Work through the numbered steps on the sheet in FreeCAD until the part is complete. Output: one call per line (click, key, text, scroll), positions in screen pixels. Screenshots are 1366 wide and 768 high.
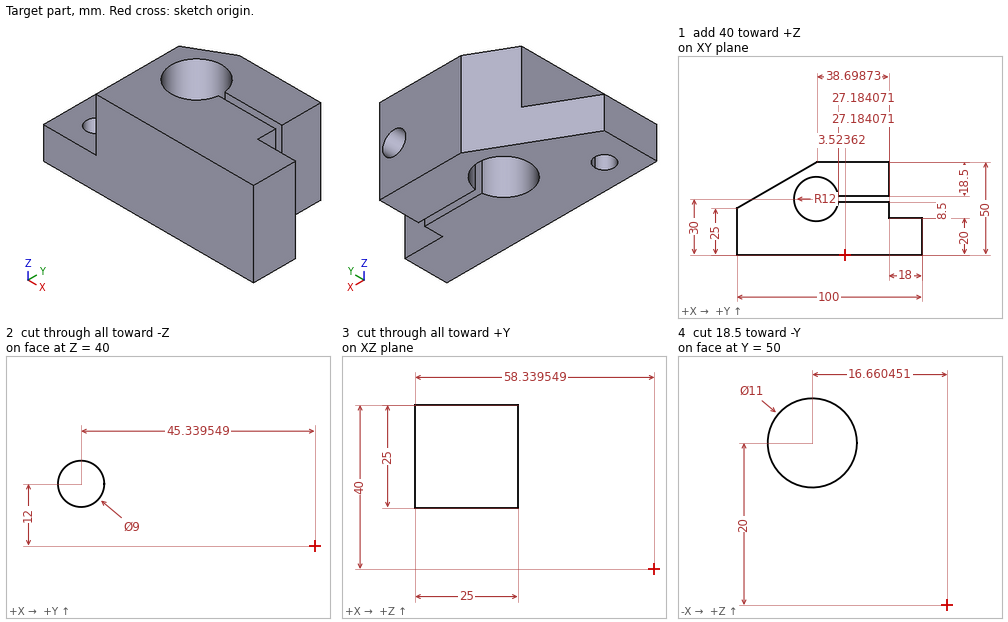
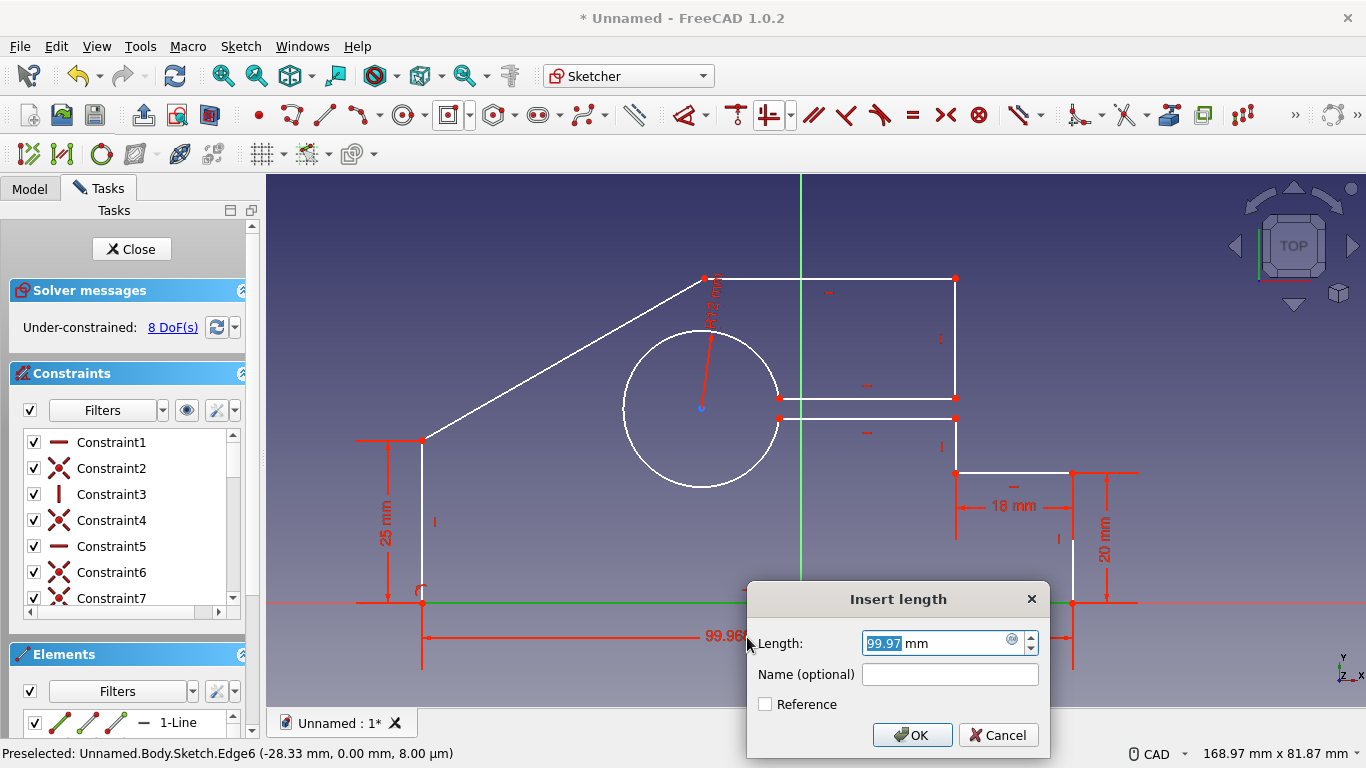
text(100)
key(Return)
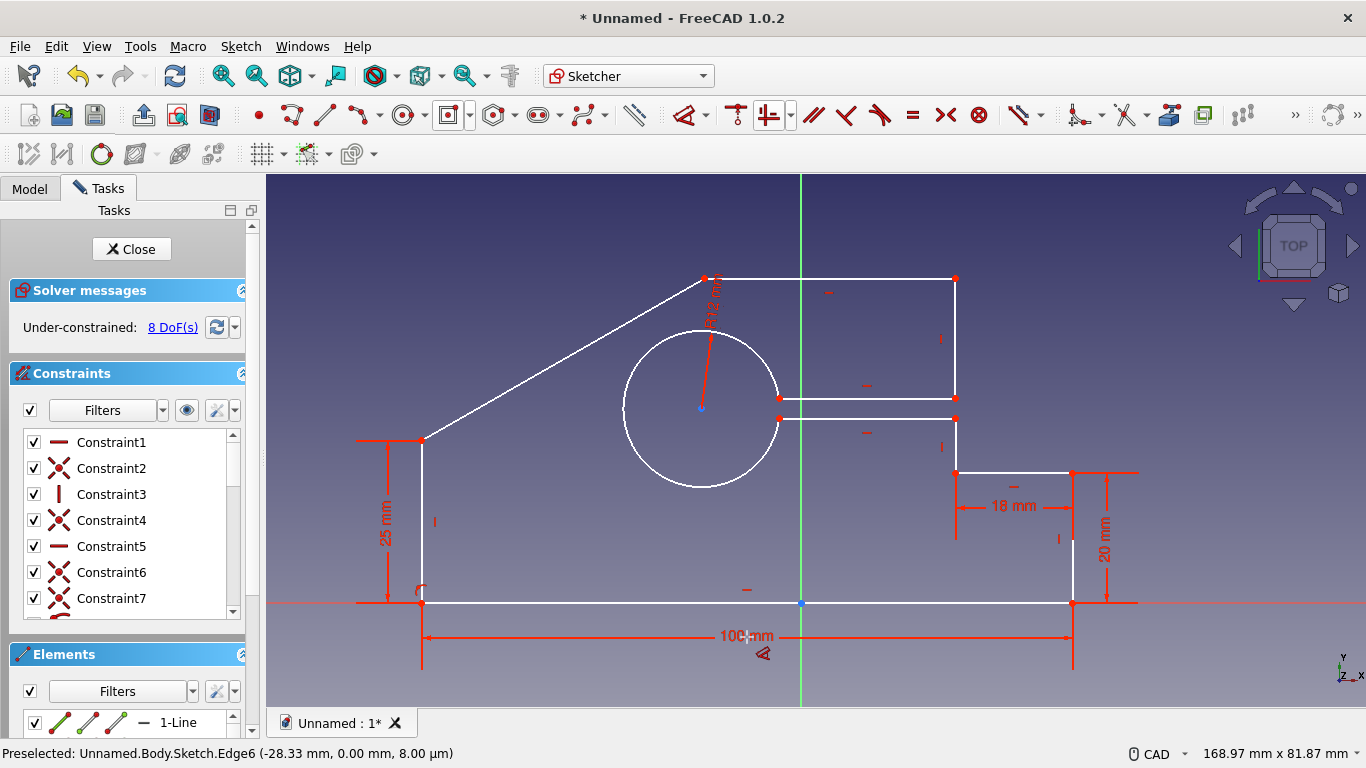
click(956, 457)
click(990, 446)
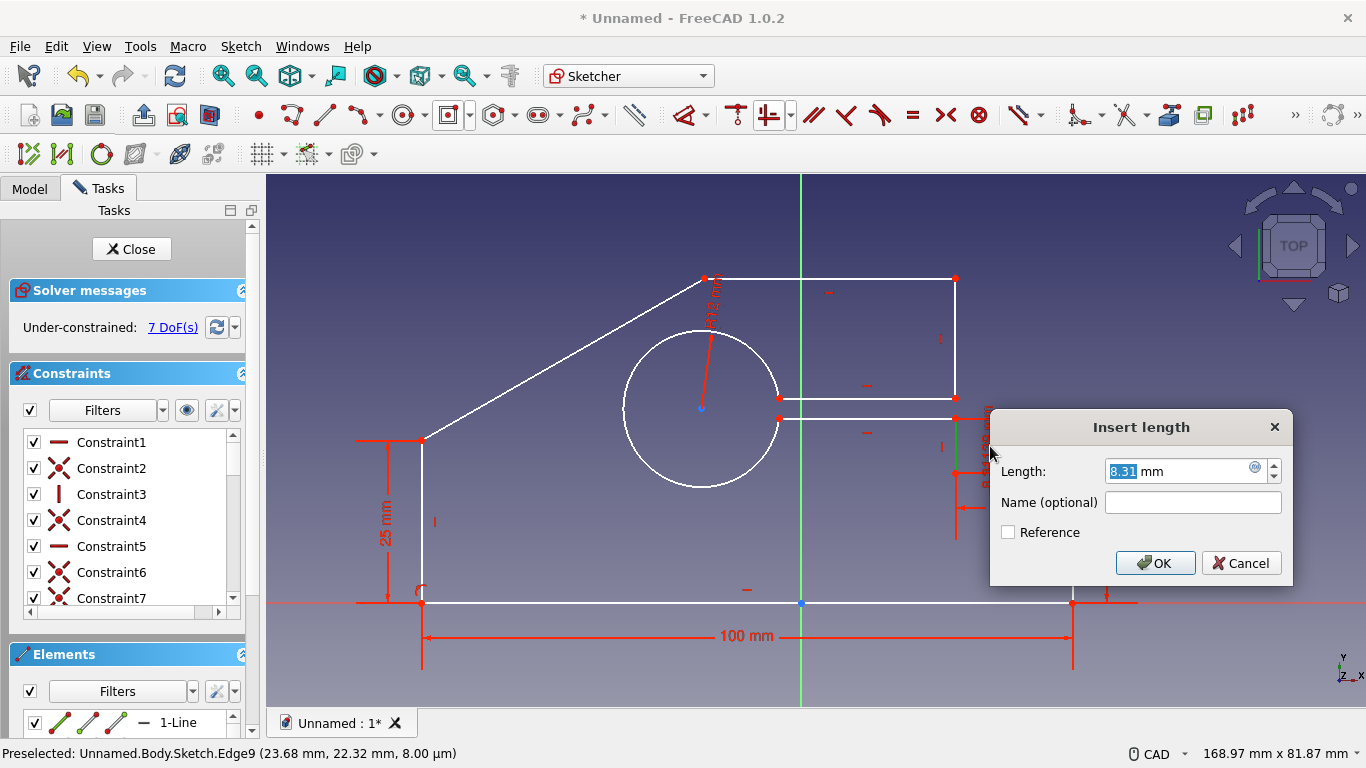
text(8.5)
key(Return)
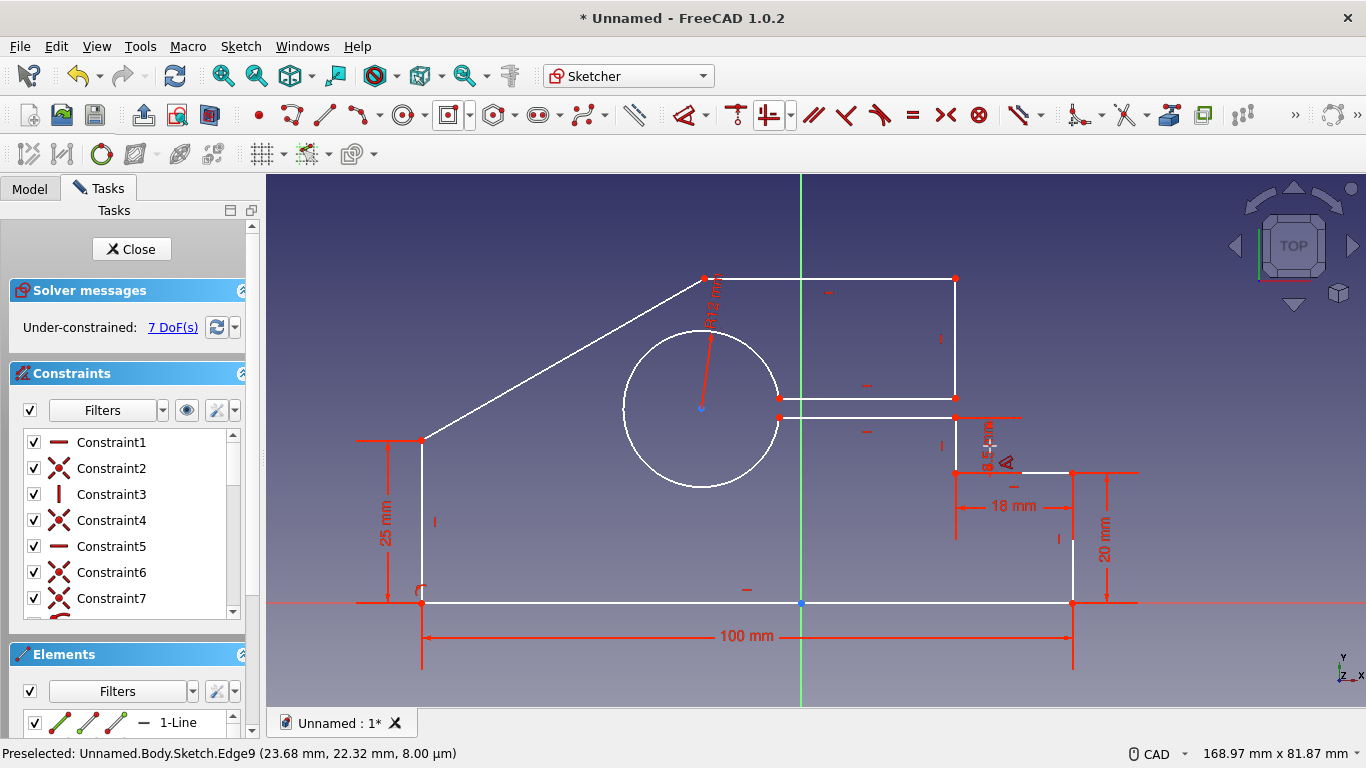
click(955, 279)
click(989, 367)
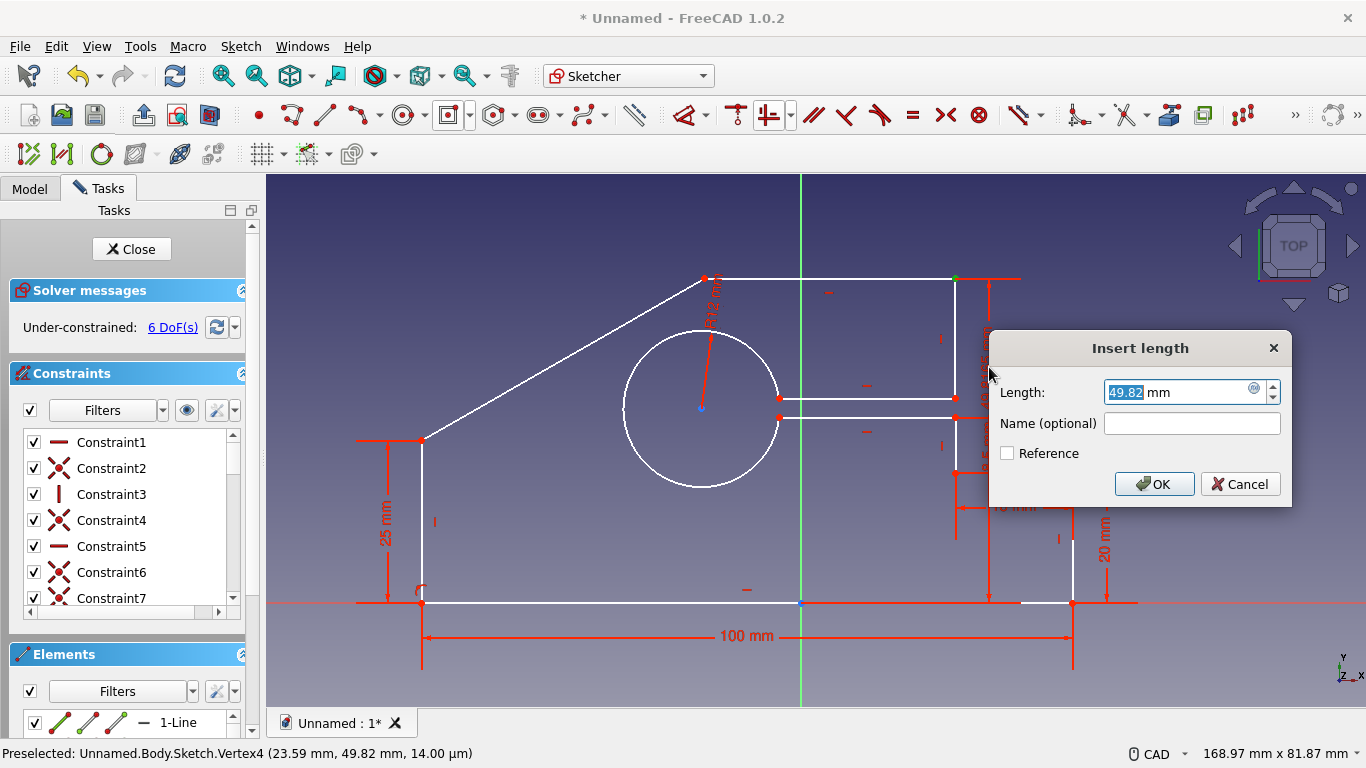
text(50)
key(Return)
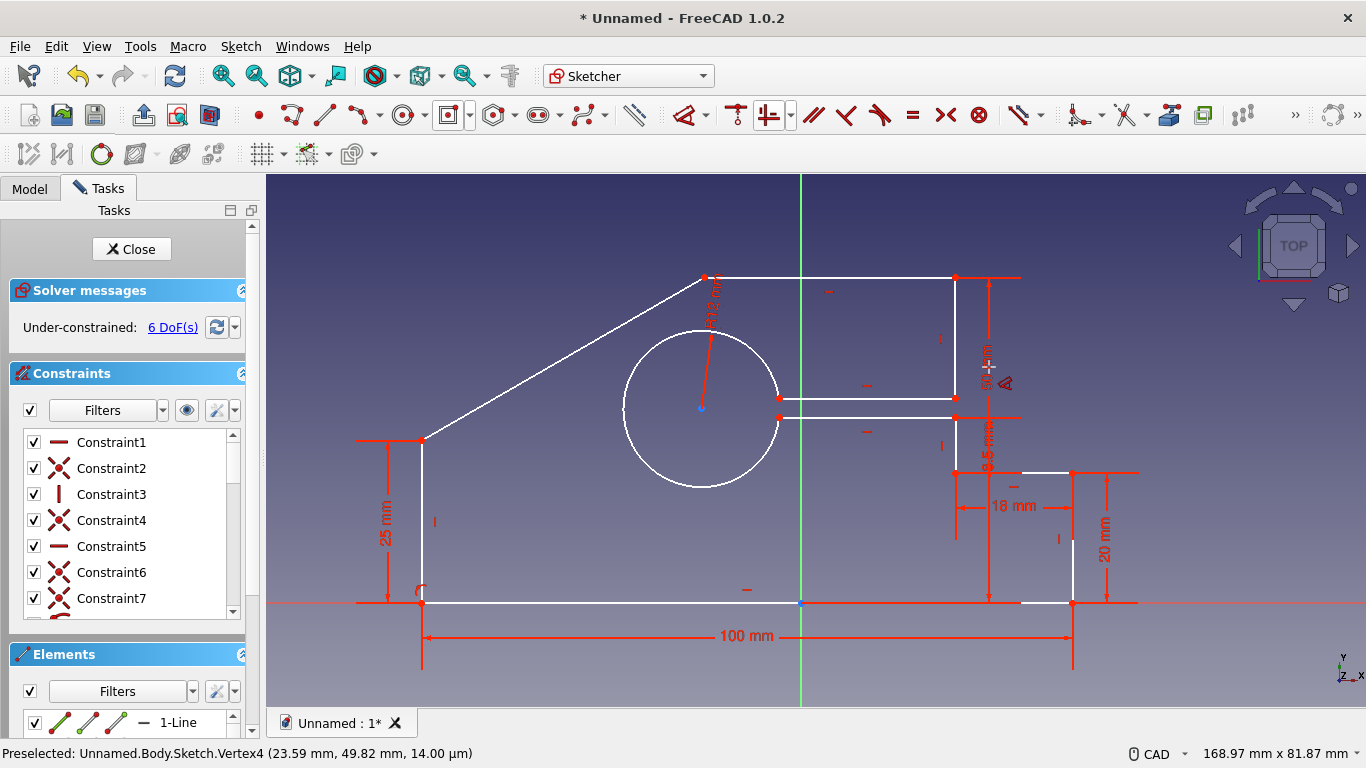
click(702, 409)
click(835, 506)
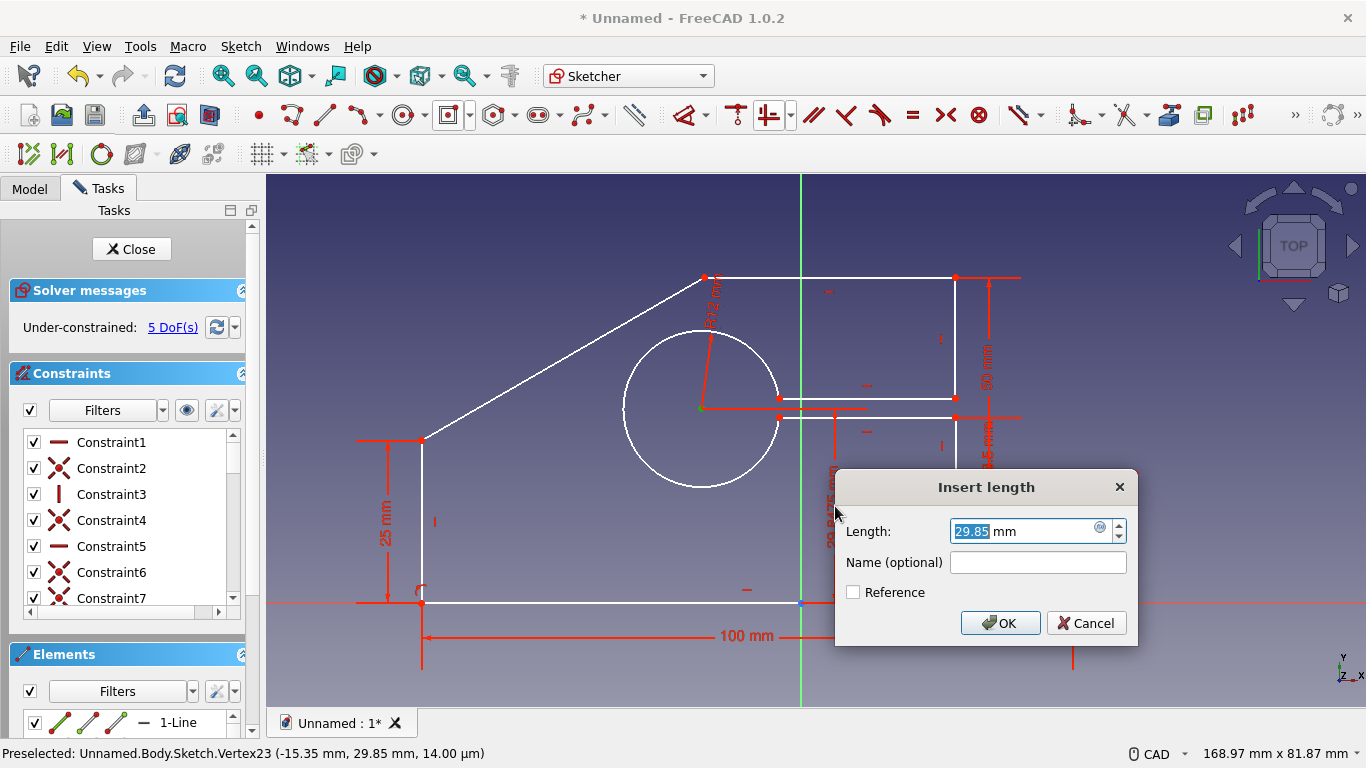
text(30)
key(Return)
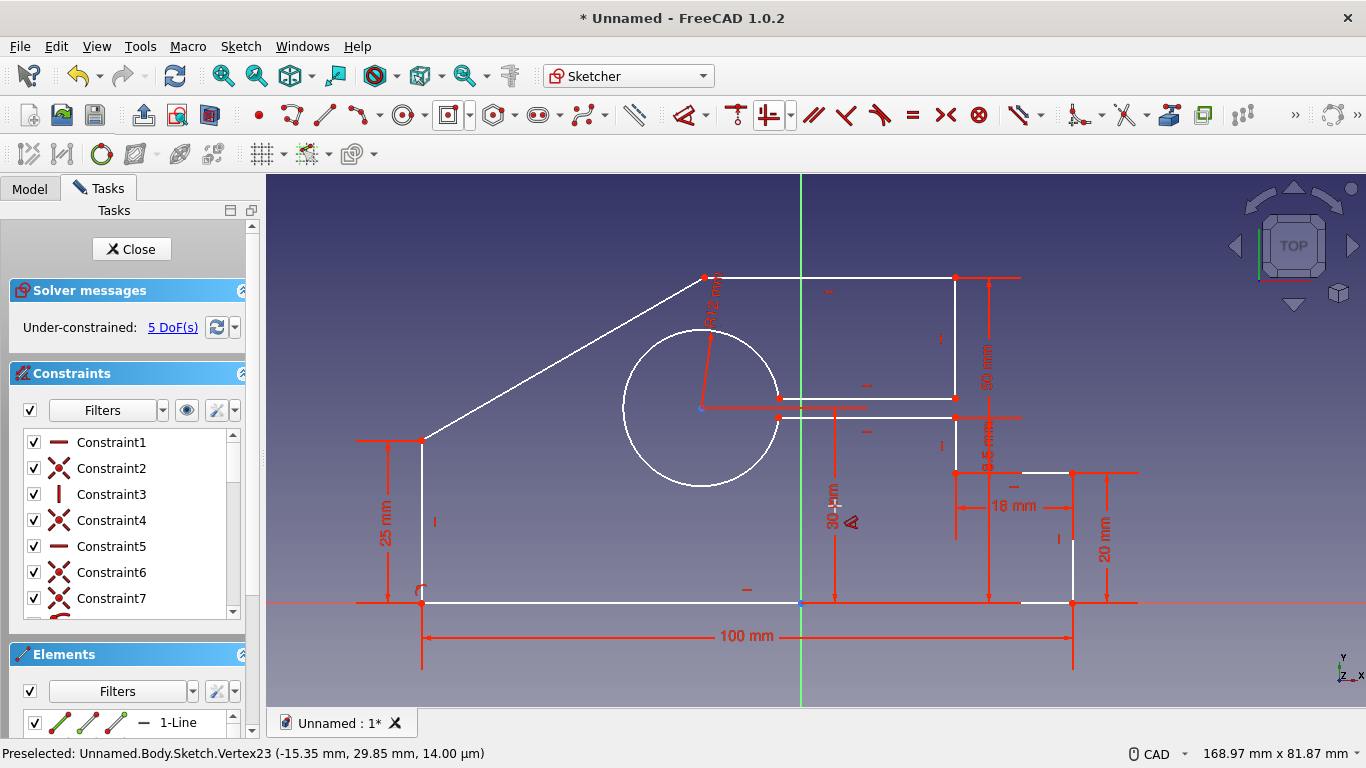
click(955, 363)
click(989, 338)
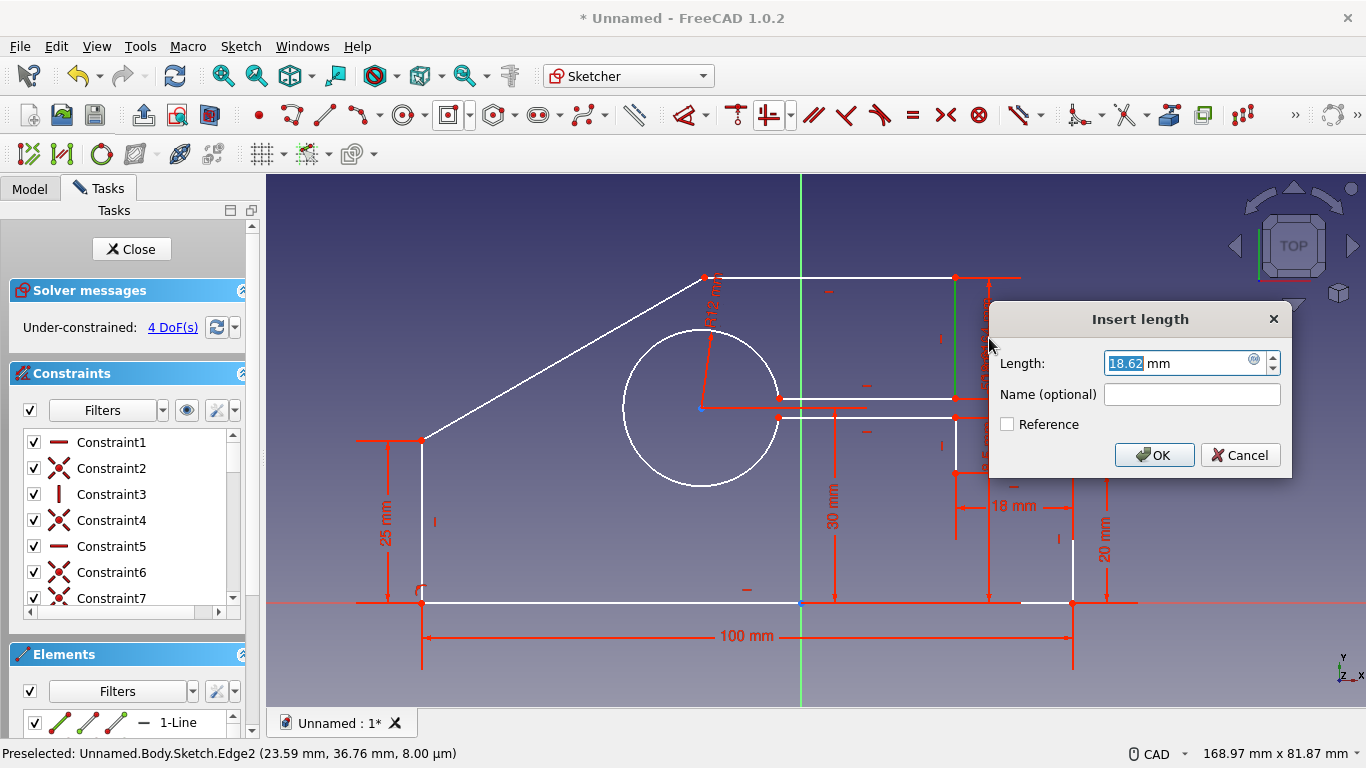
text(18.5)
key(Return)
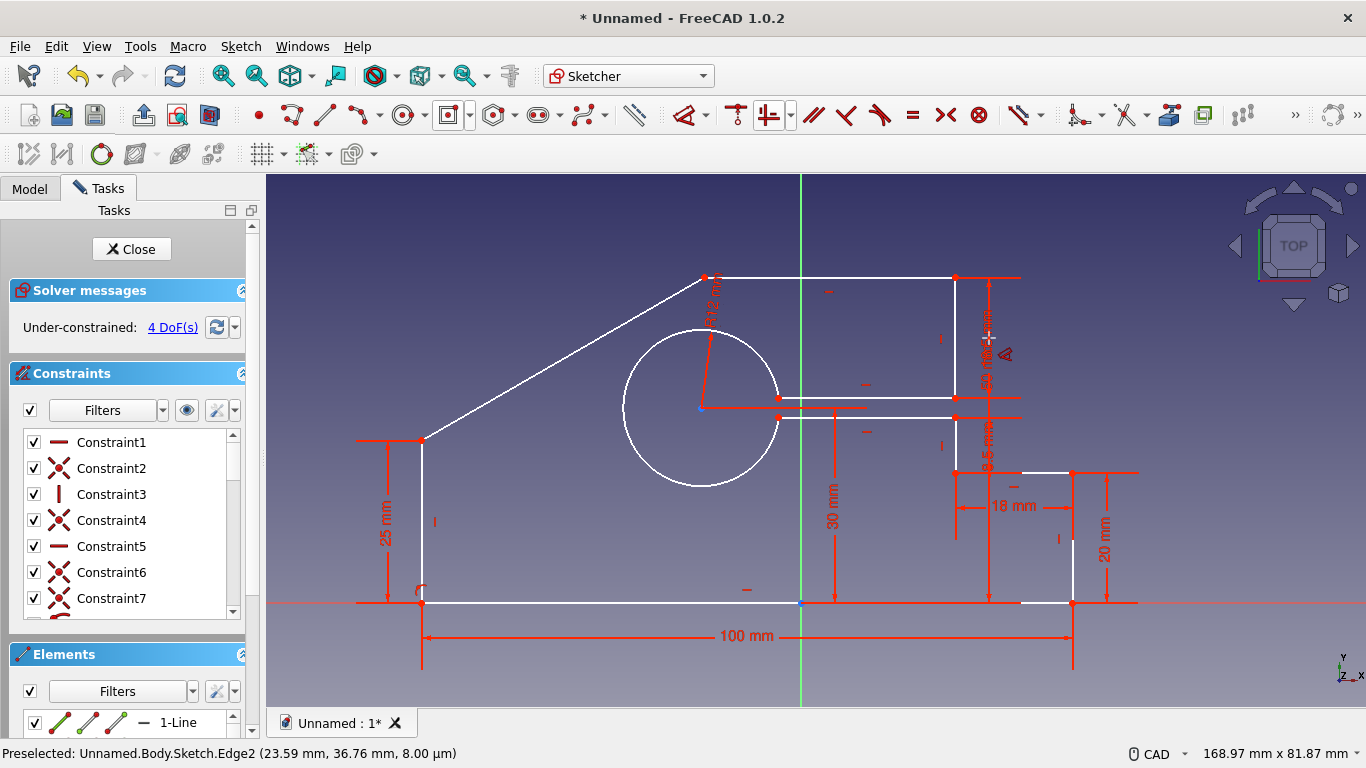
click(880, 278)
click(829, 244)